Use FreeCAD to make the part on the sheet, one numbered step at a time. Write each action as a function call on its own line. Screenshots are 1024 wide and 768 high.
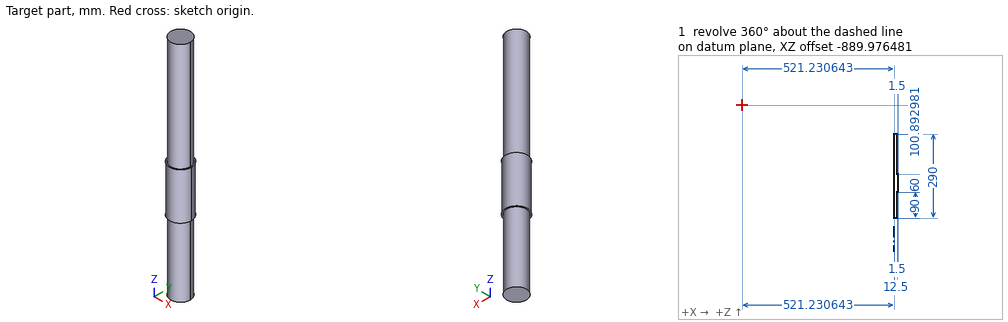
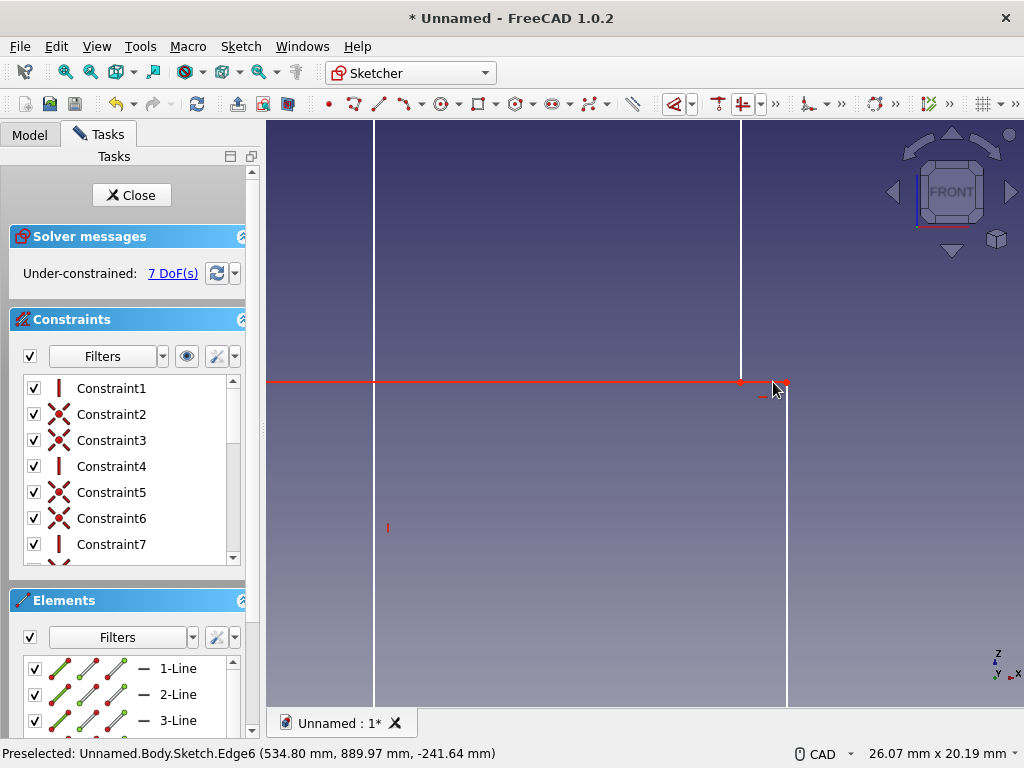
click(692, 104)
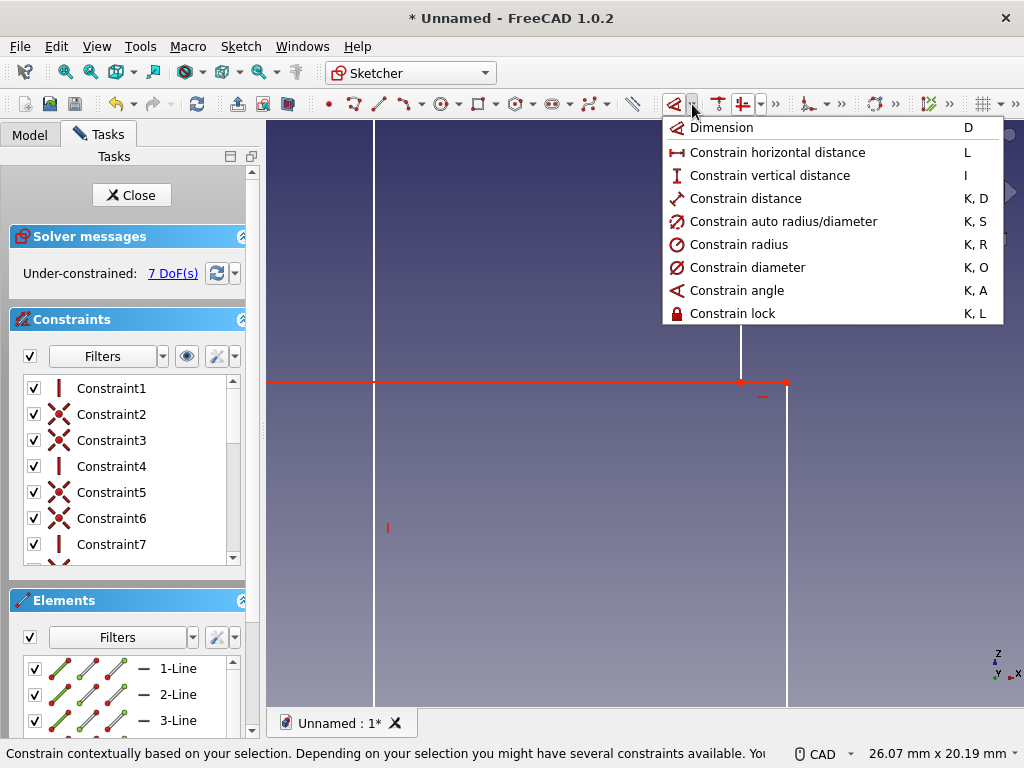
click(833, 152)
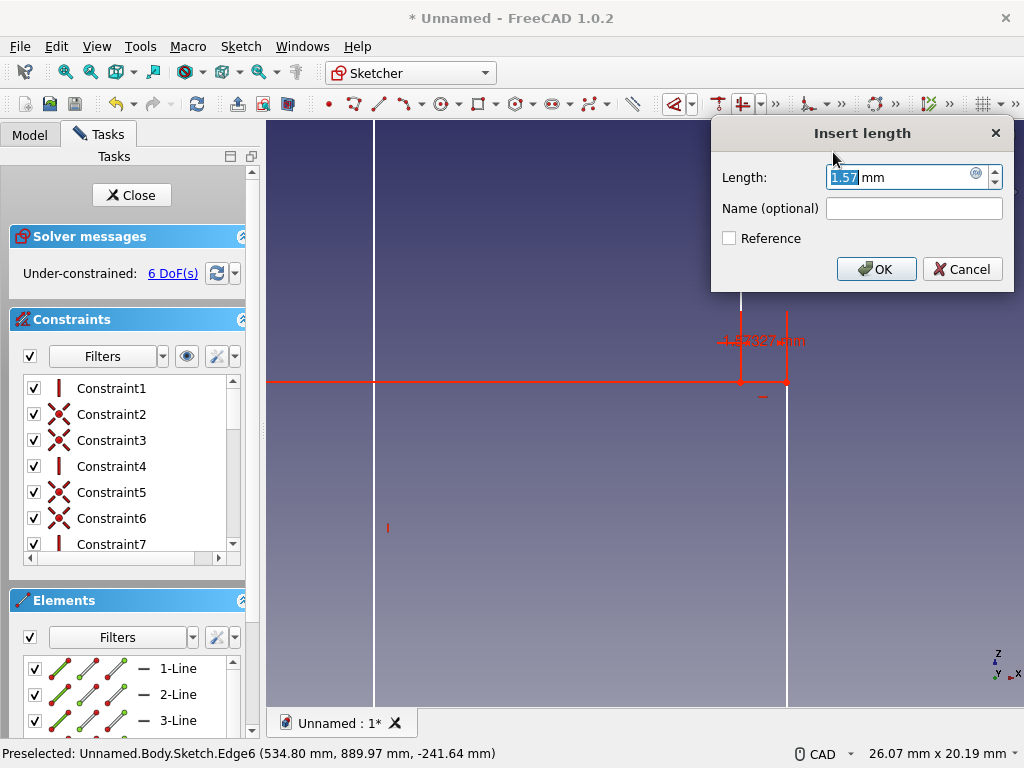
text(1.5)
key(Return)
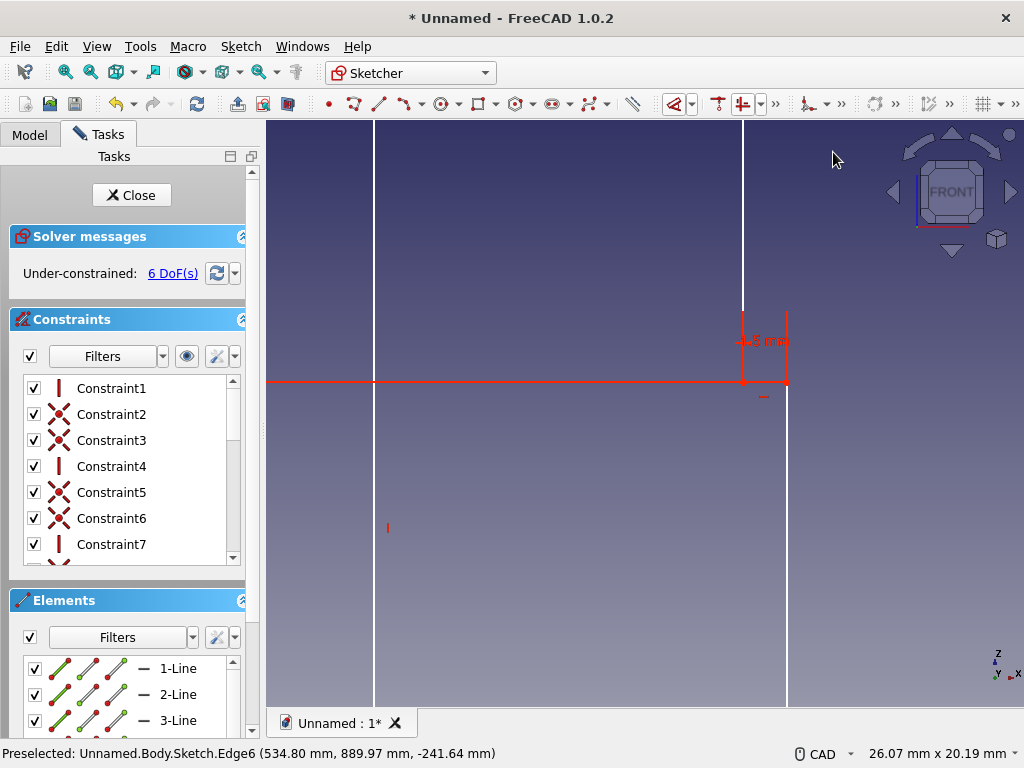
scroll(789, 405, down, 18)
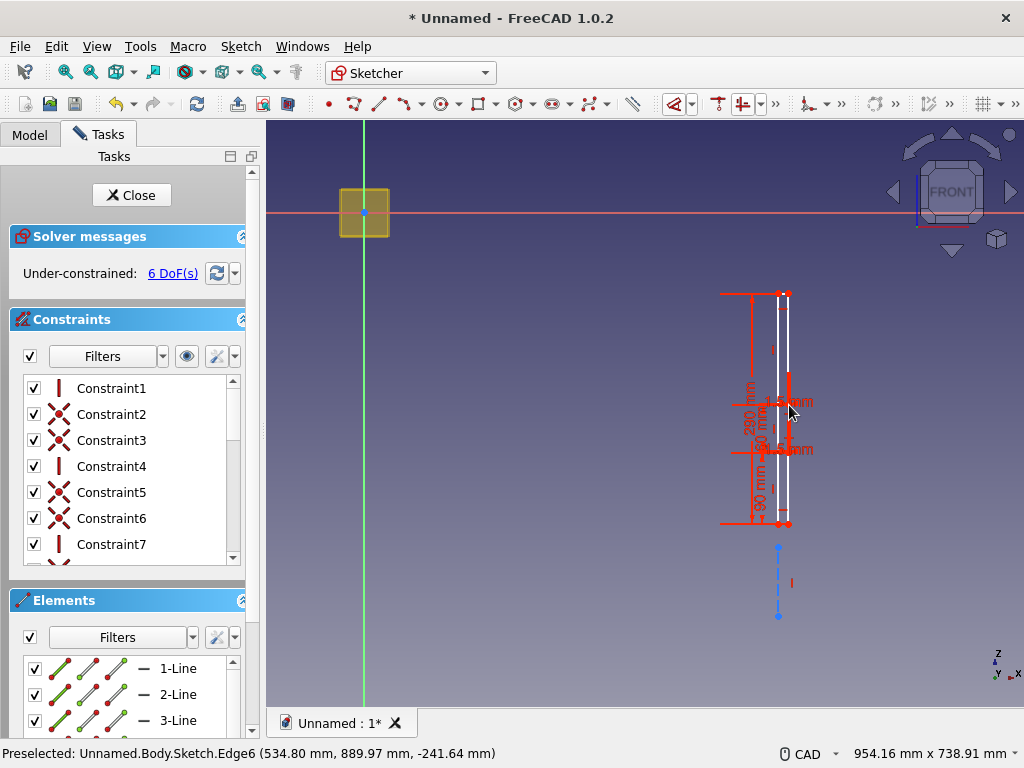
scroll(781, 524, up, 8)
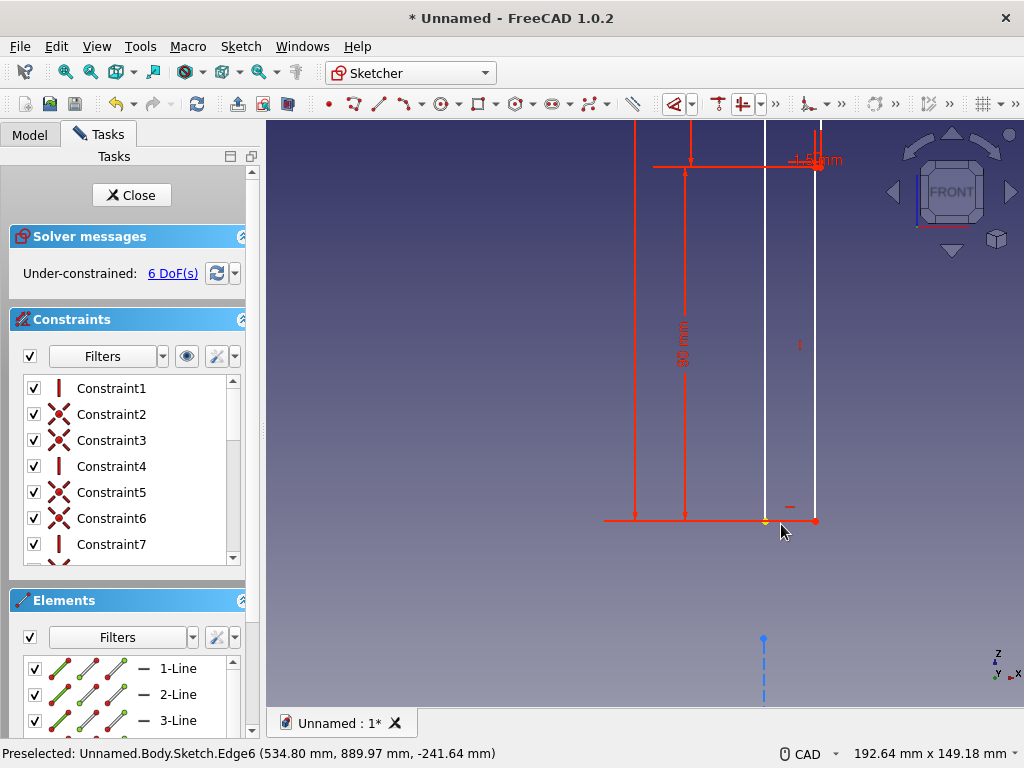
click(780, 521)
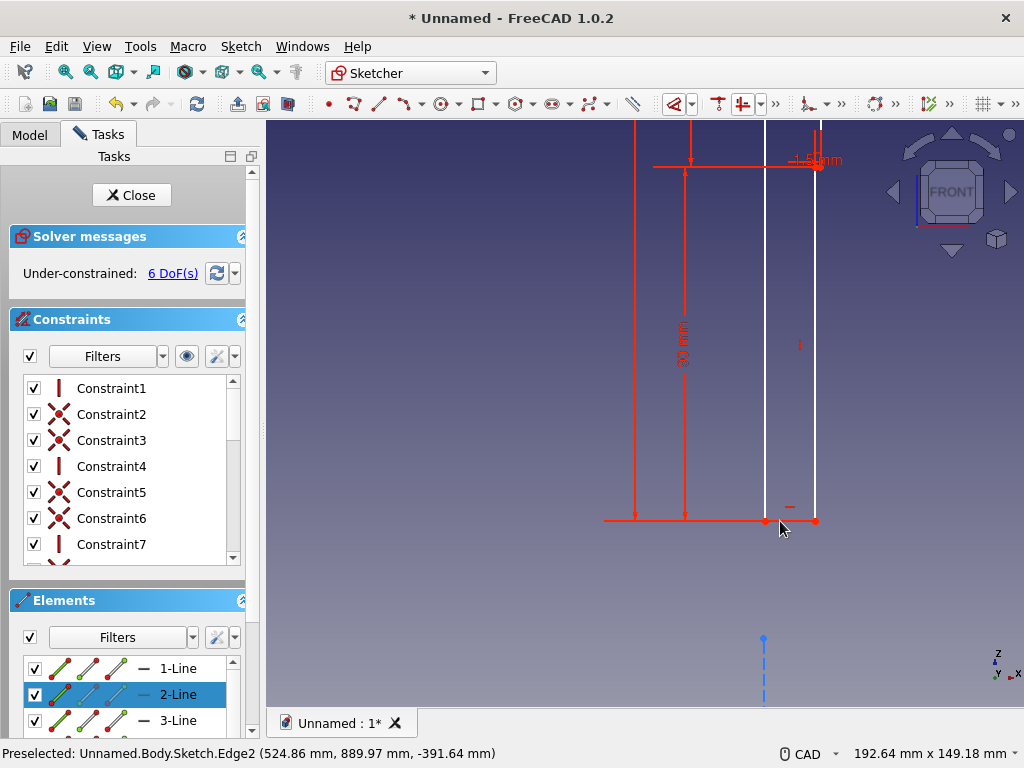
key(l)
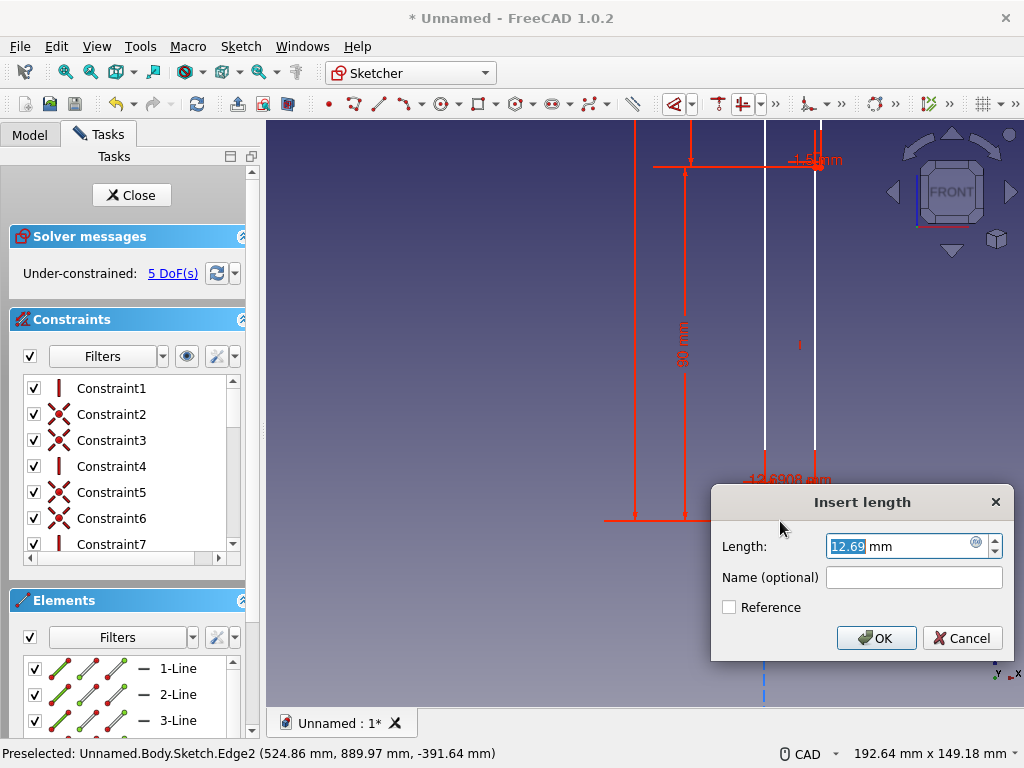
text(12.5)
key(Return)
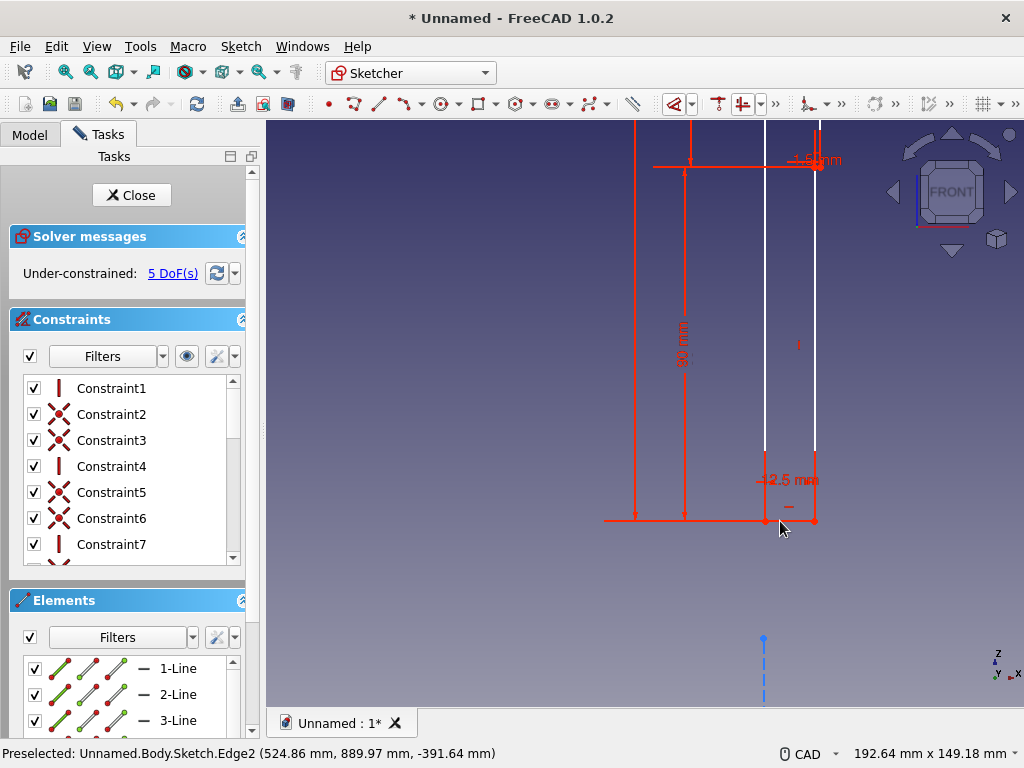
scroll(781, 524, down, 8)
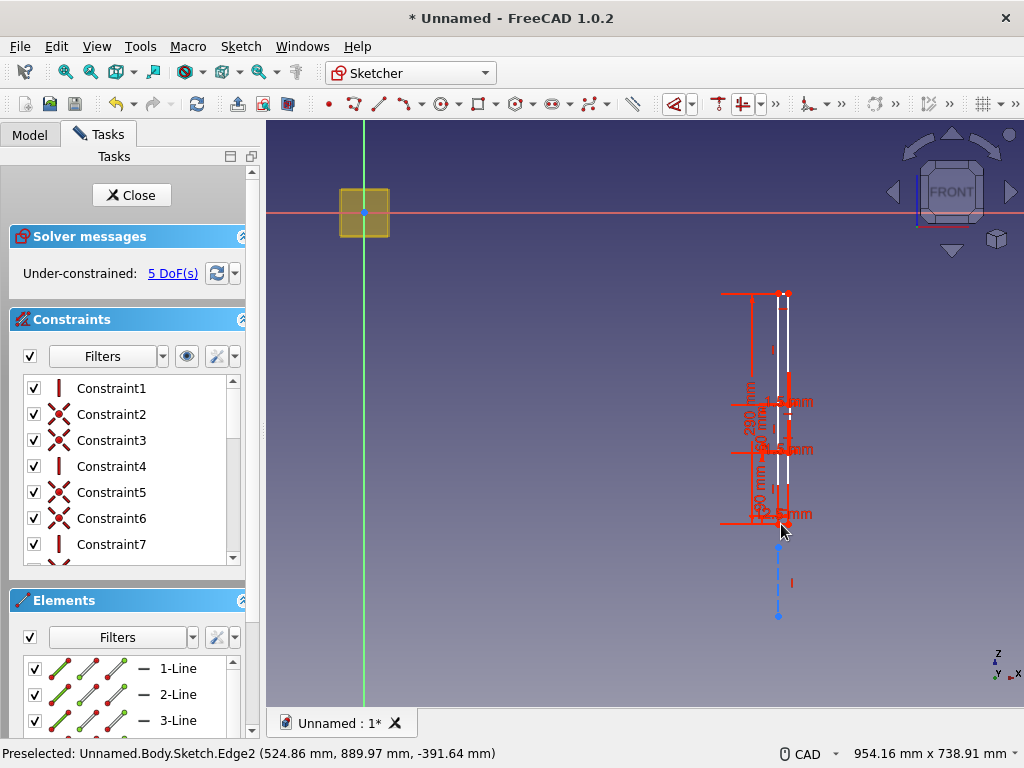
scroll(778, 294, up, 2)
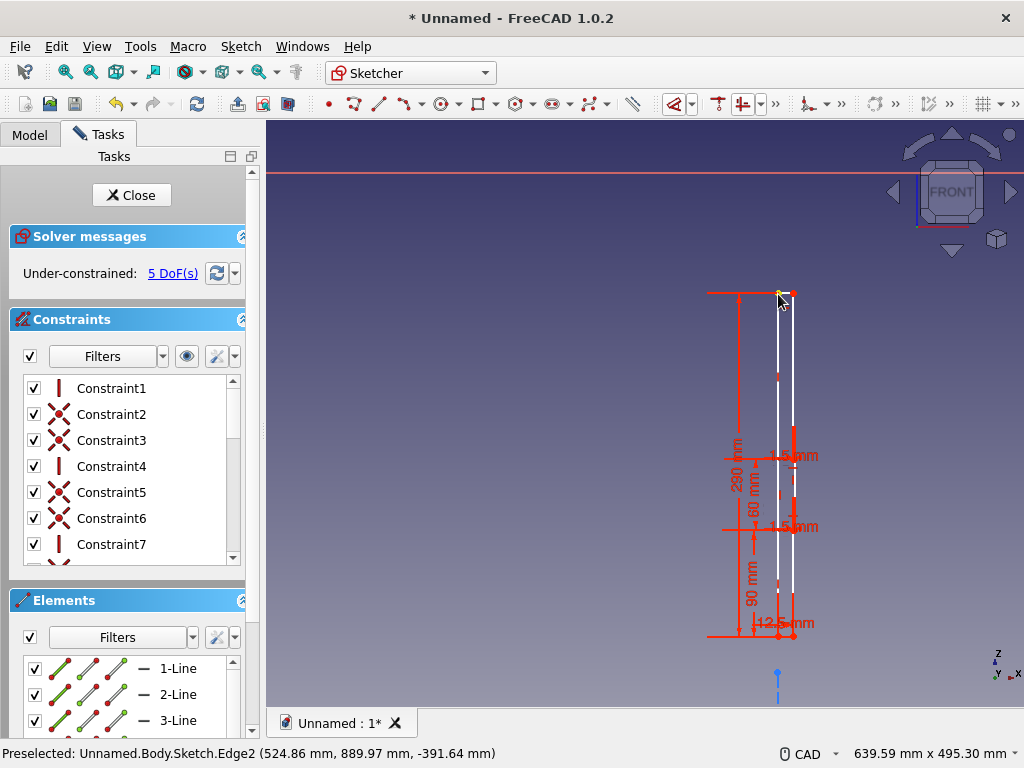
click(778, 293)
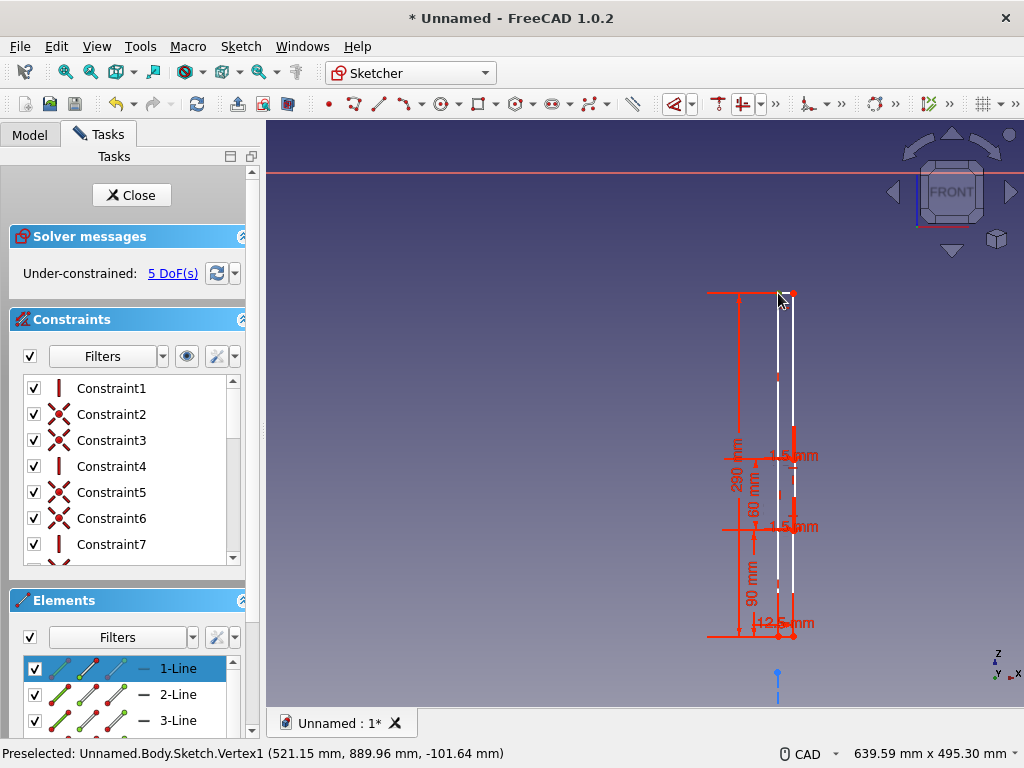
click(692, 104)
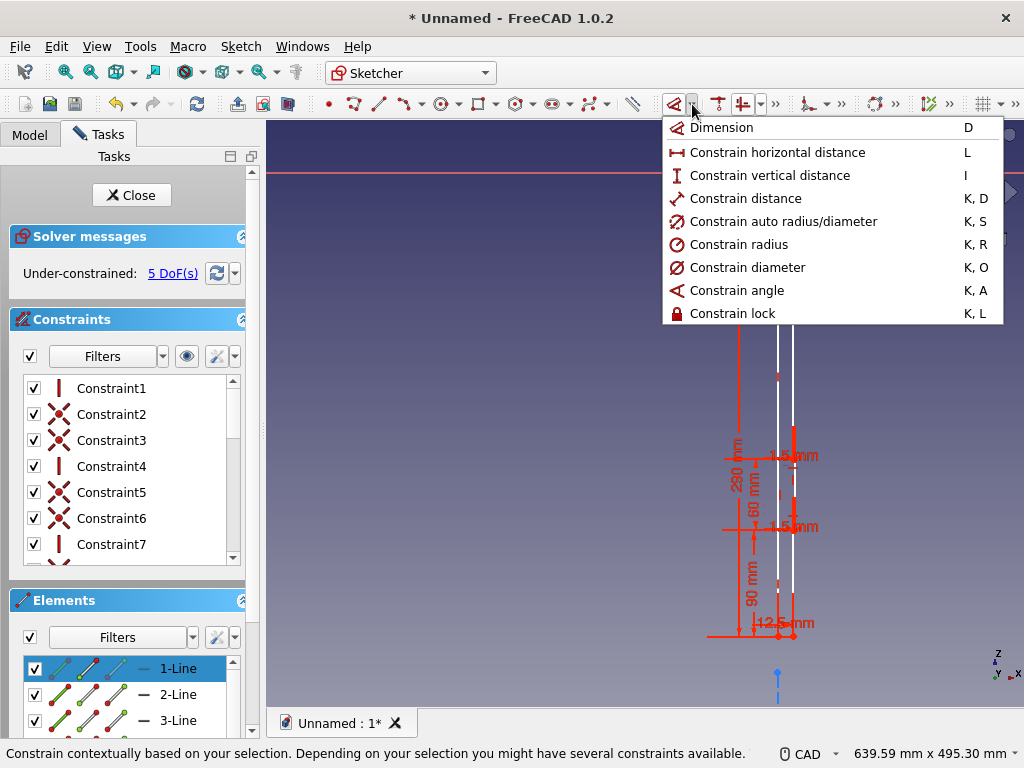
click(833, 152)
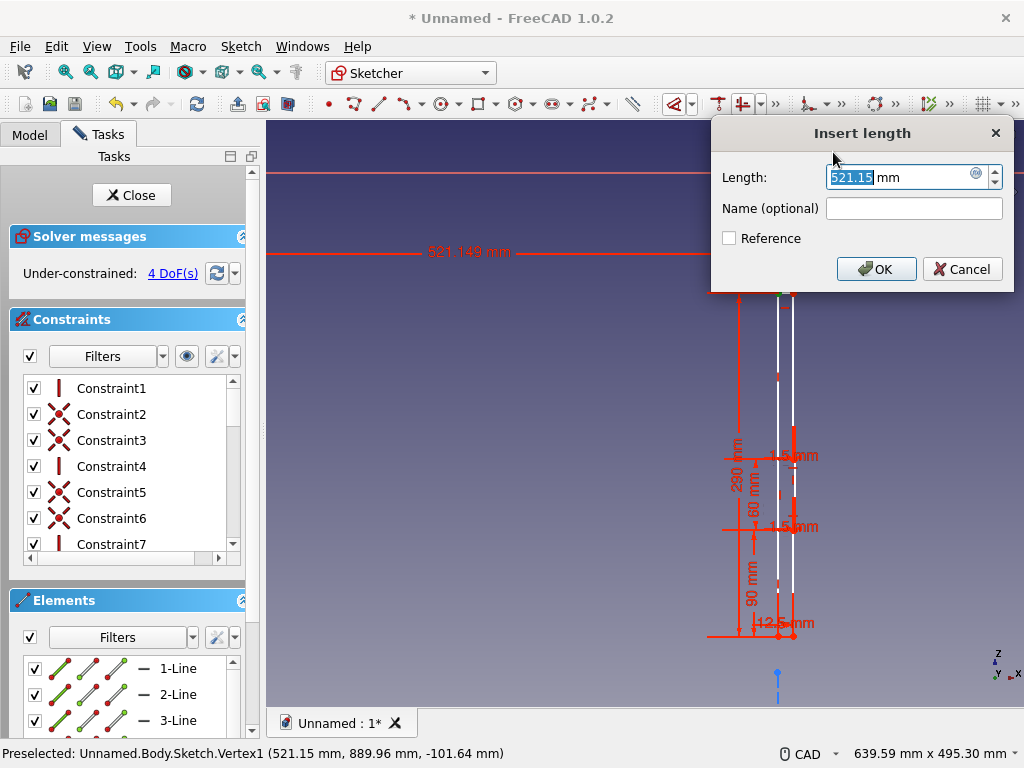
text(521.230643)
key(Return)